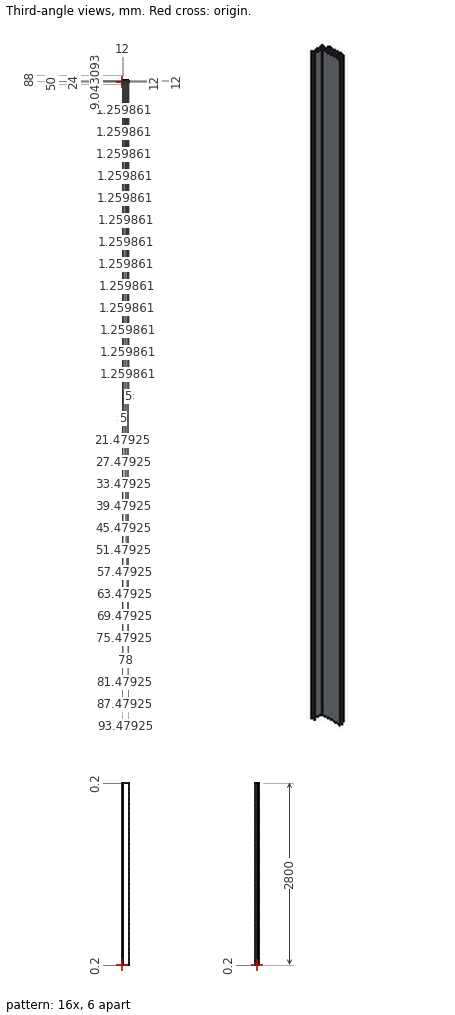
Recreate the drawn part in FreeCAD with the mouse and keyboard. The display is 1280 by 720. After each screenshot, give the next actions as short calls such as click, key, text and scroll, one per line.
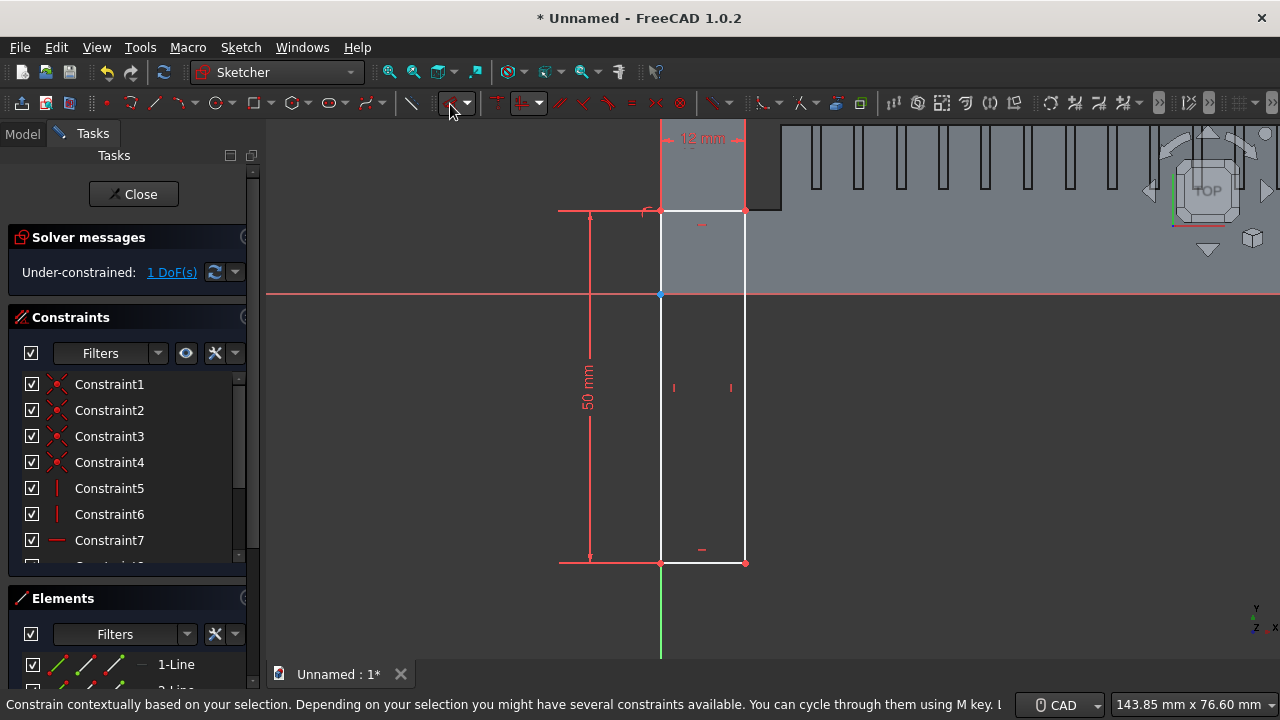
click(661, 211)
click(627, 253)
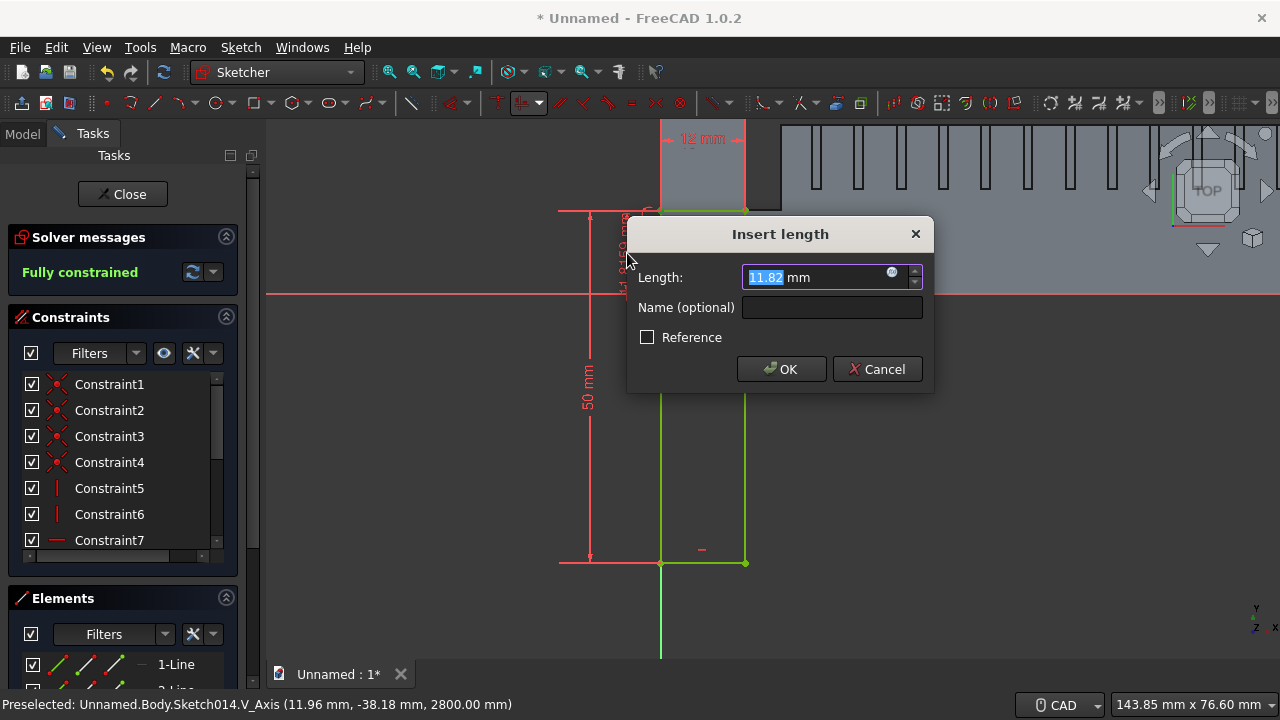
text(12)
key(Return)
key(Escape)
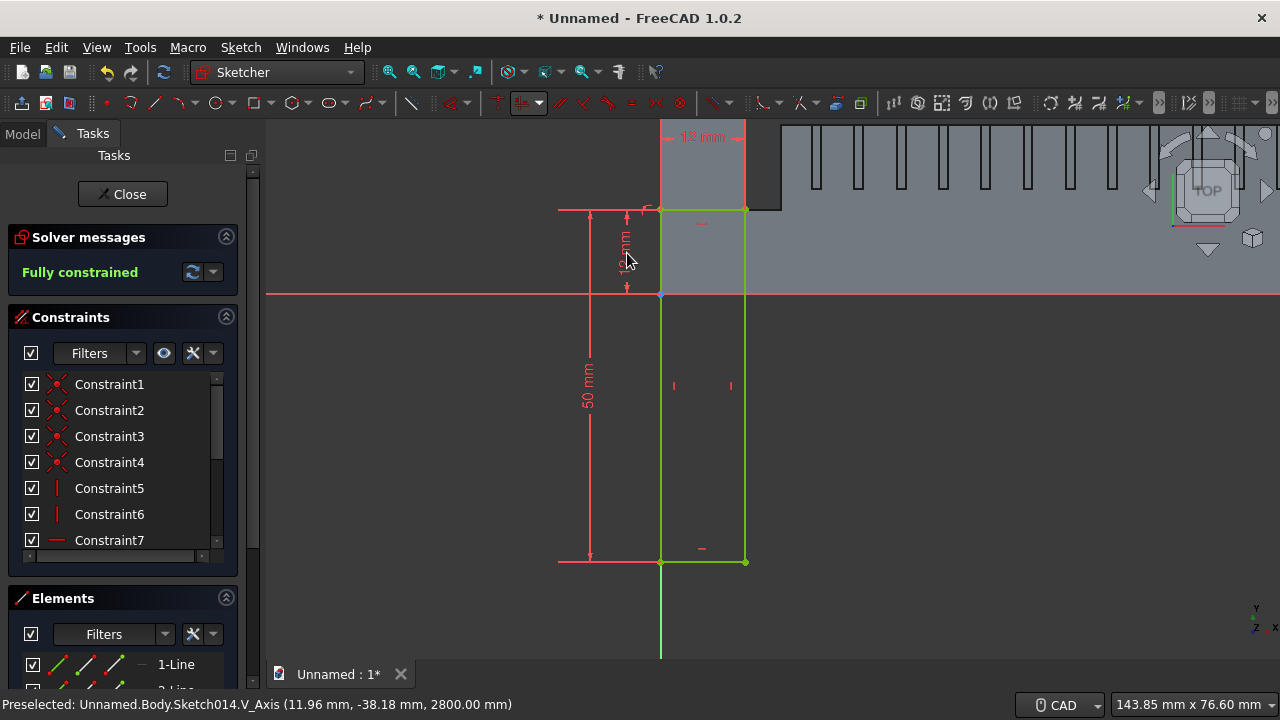
click(123, 194)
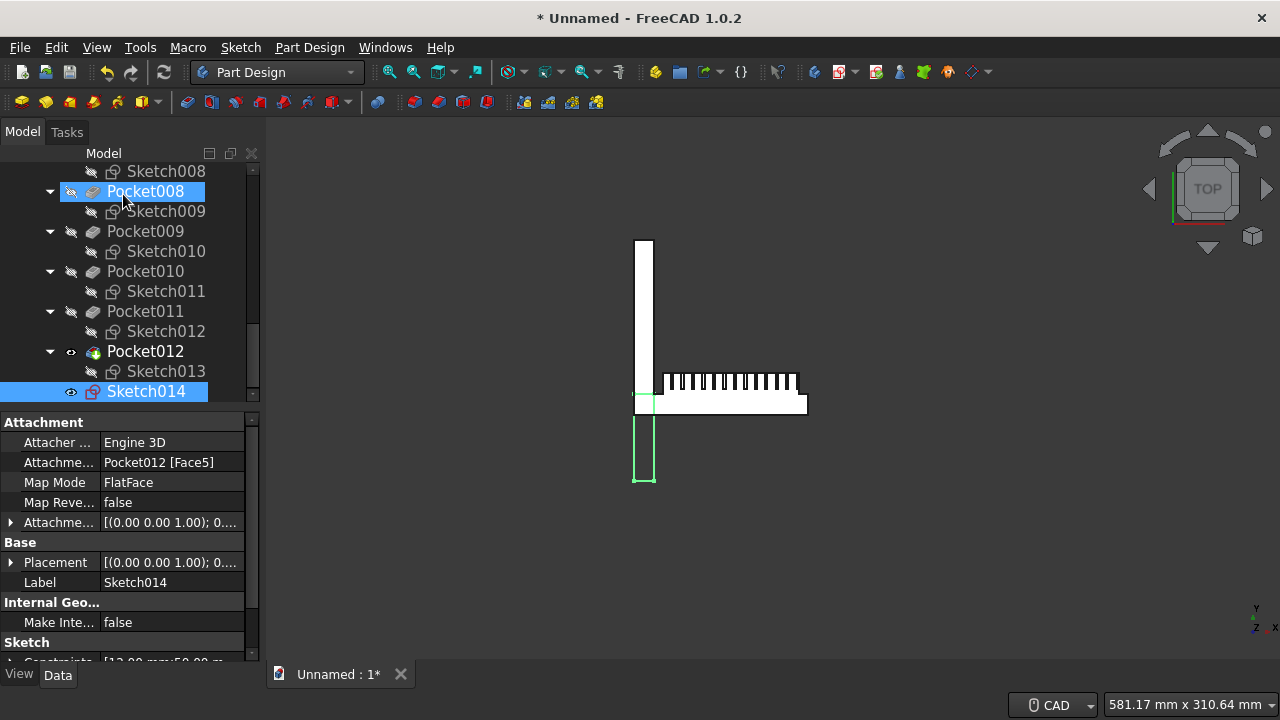
click(22, 102)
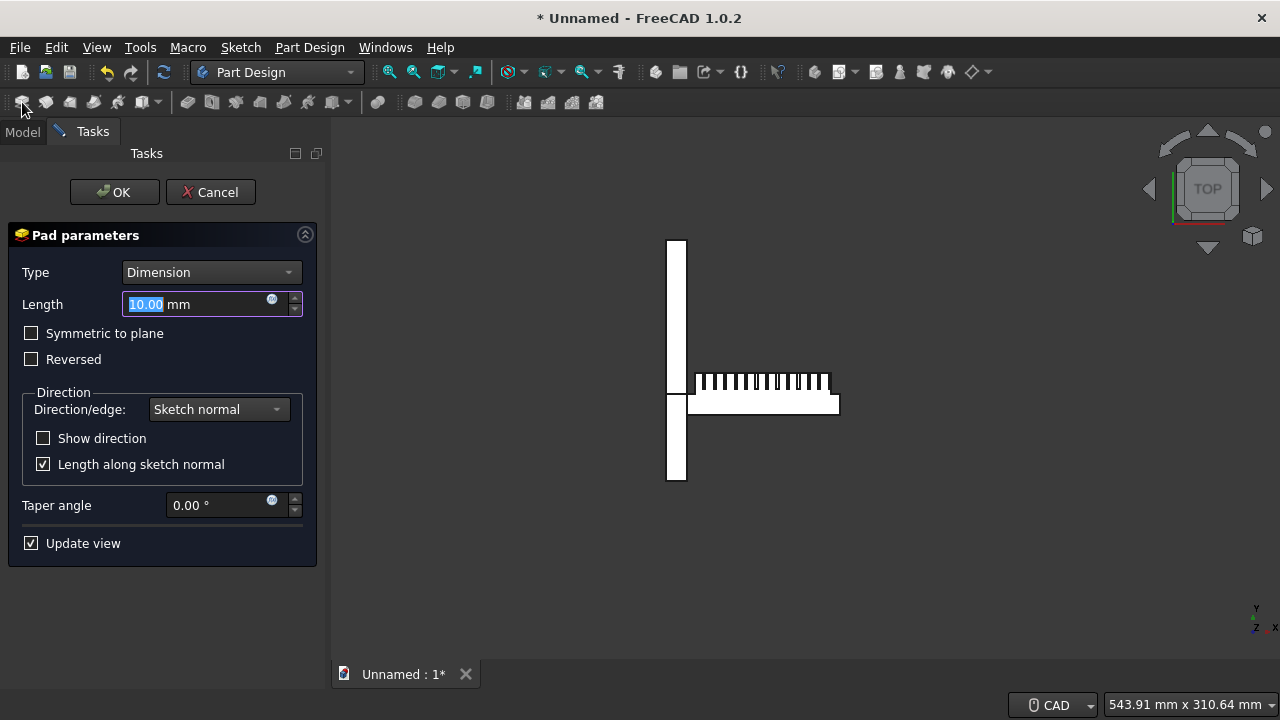
text(2800)
key(Tab)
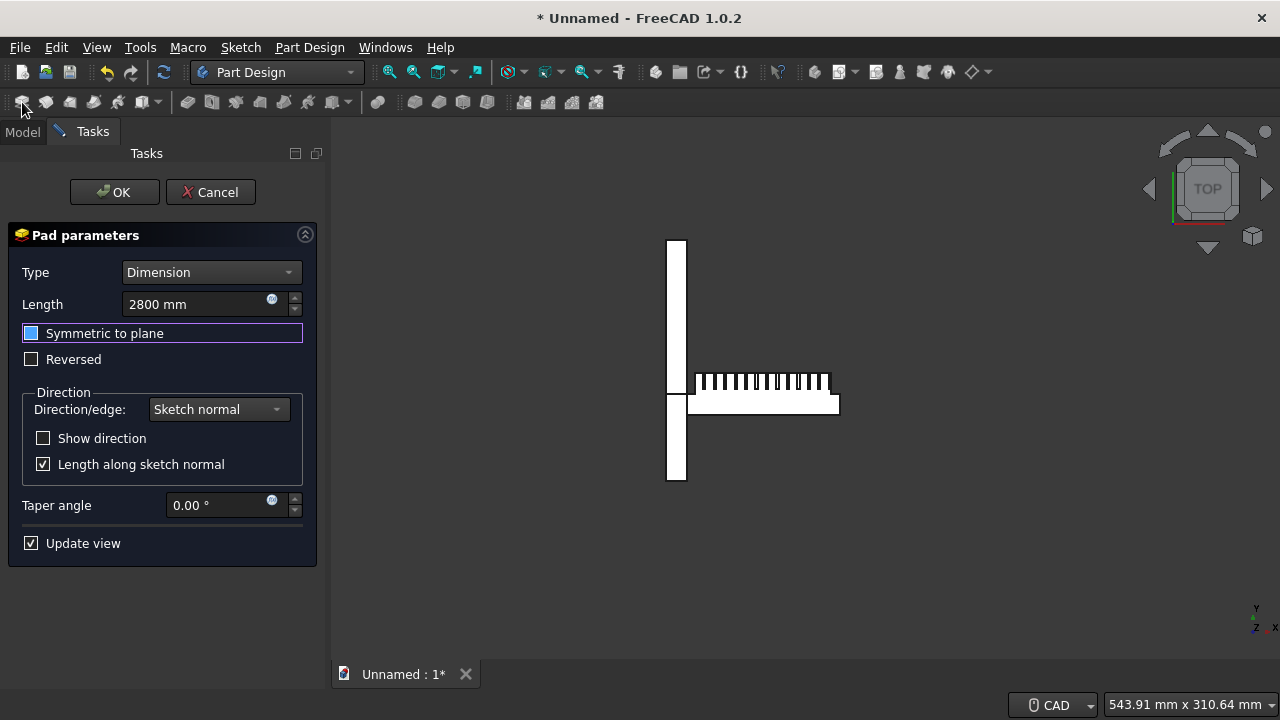
click(30, 359)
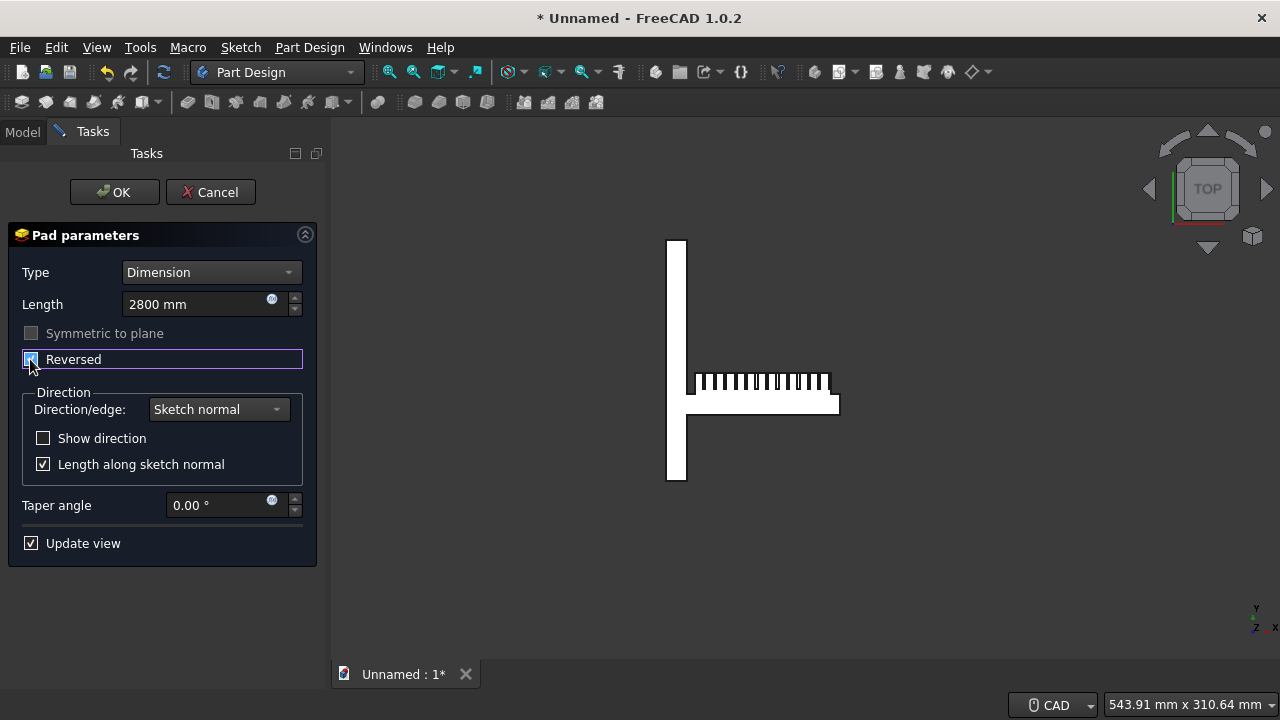
click(115, 192)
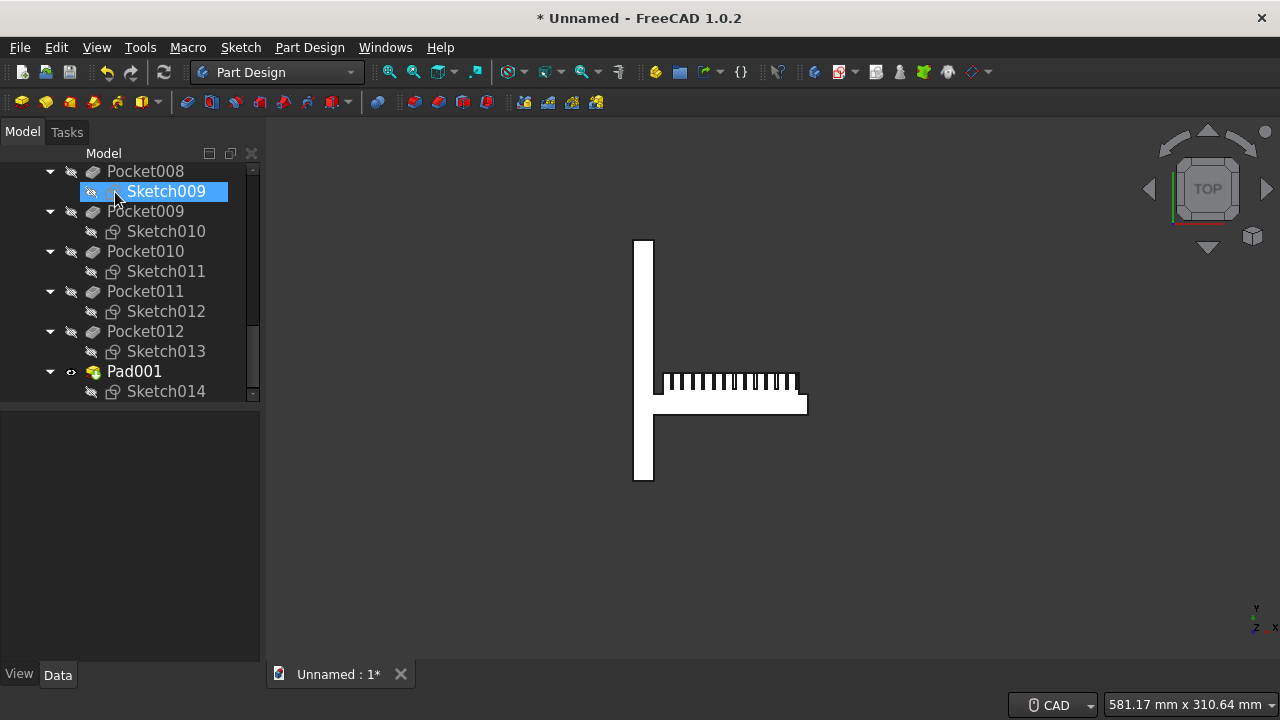
click(390, 72)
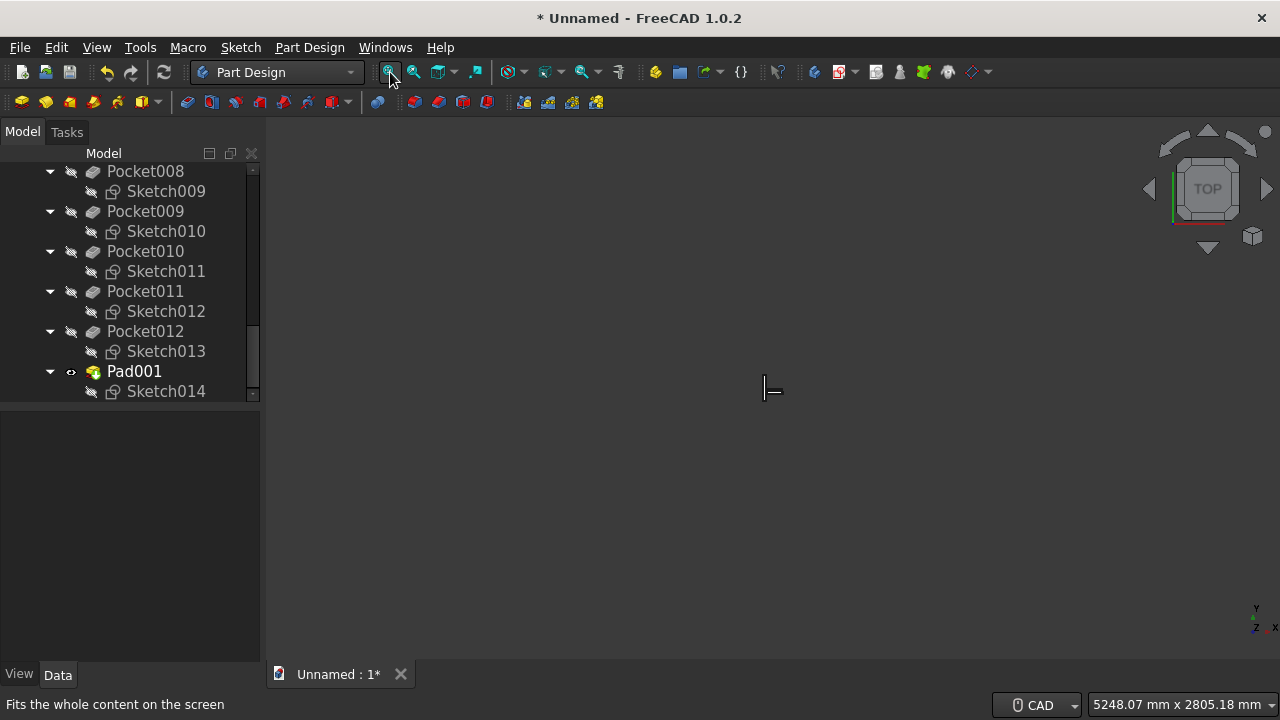
scroll(765, 391, up, 13)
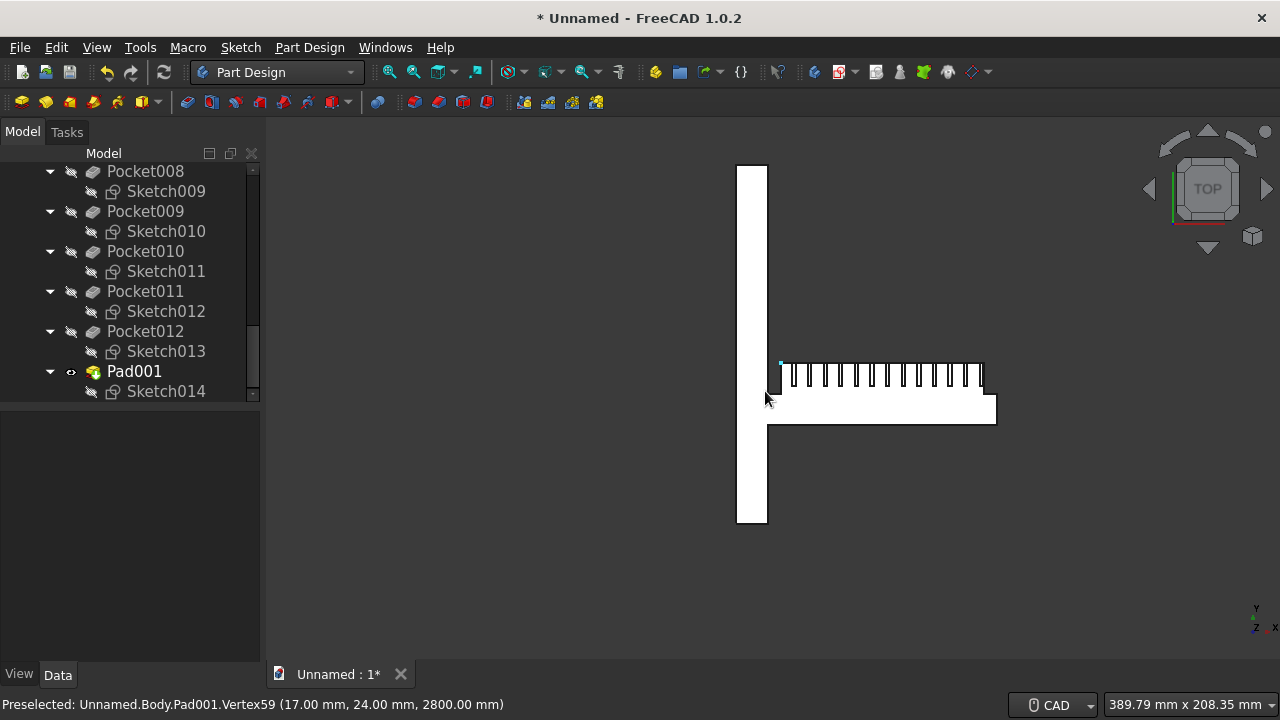
click(755, 395)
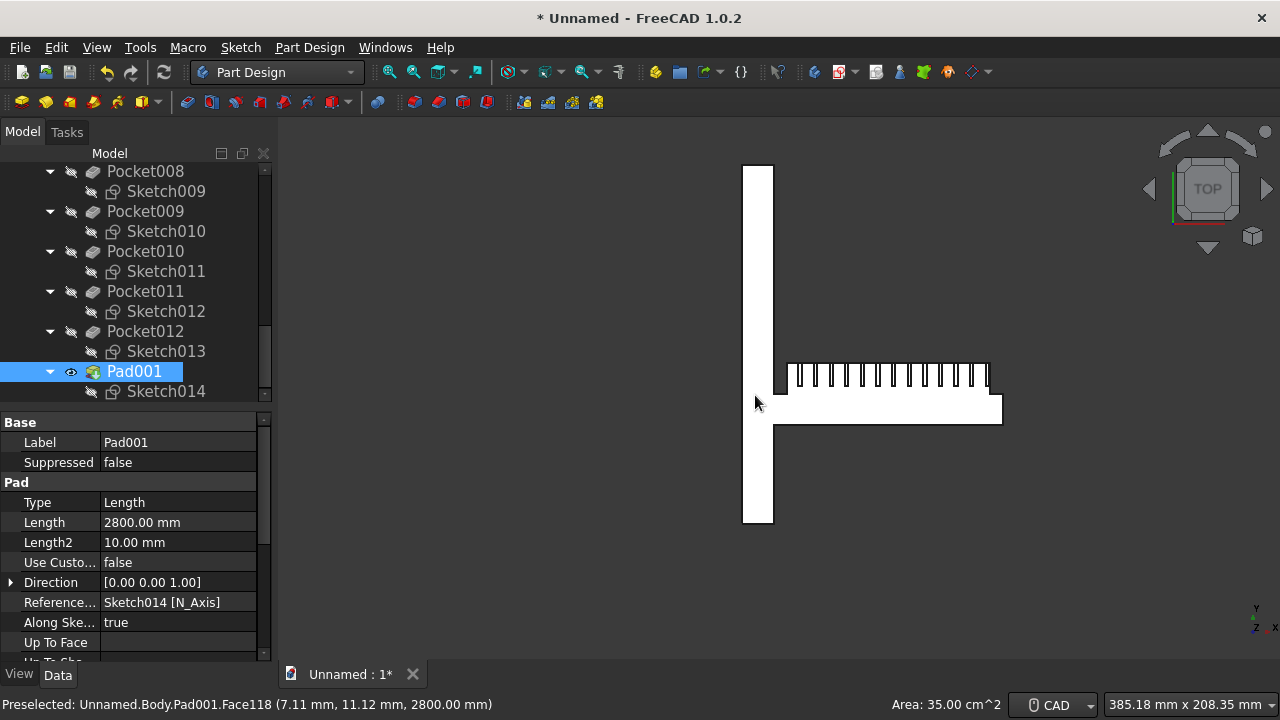
click(840, 72)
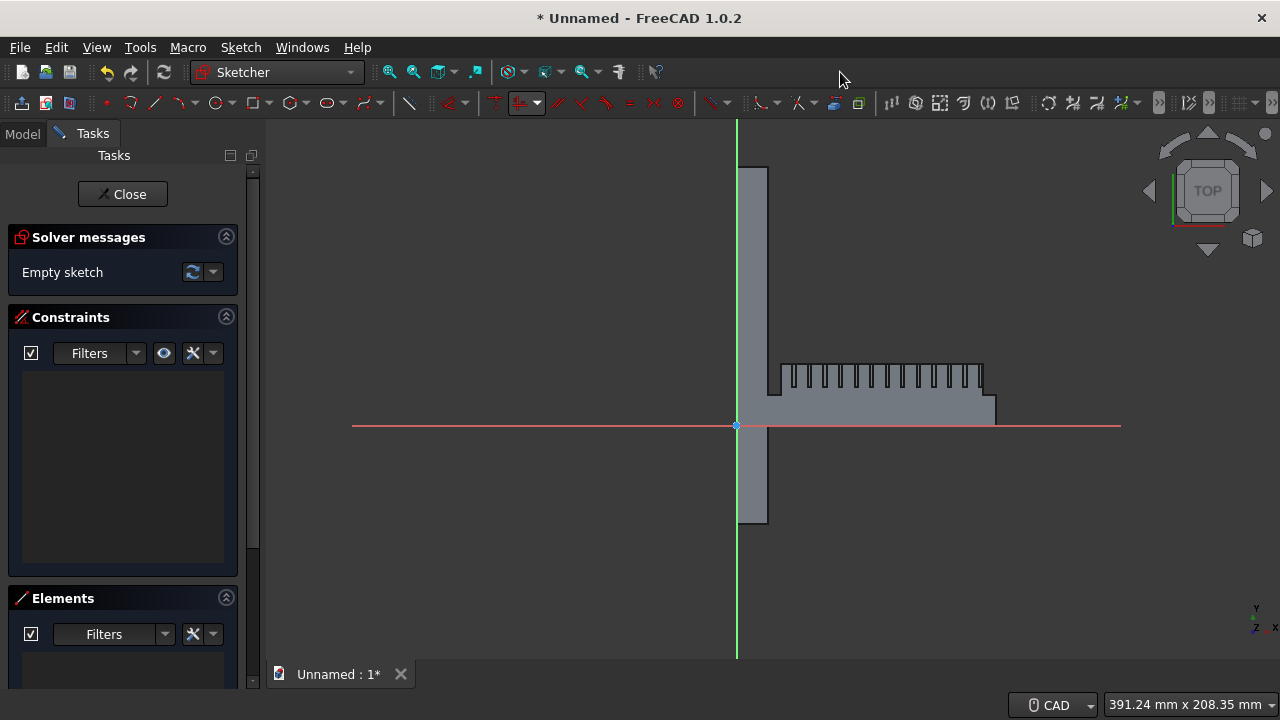
scroll(489, 631, down, 1)